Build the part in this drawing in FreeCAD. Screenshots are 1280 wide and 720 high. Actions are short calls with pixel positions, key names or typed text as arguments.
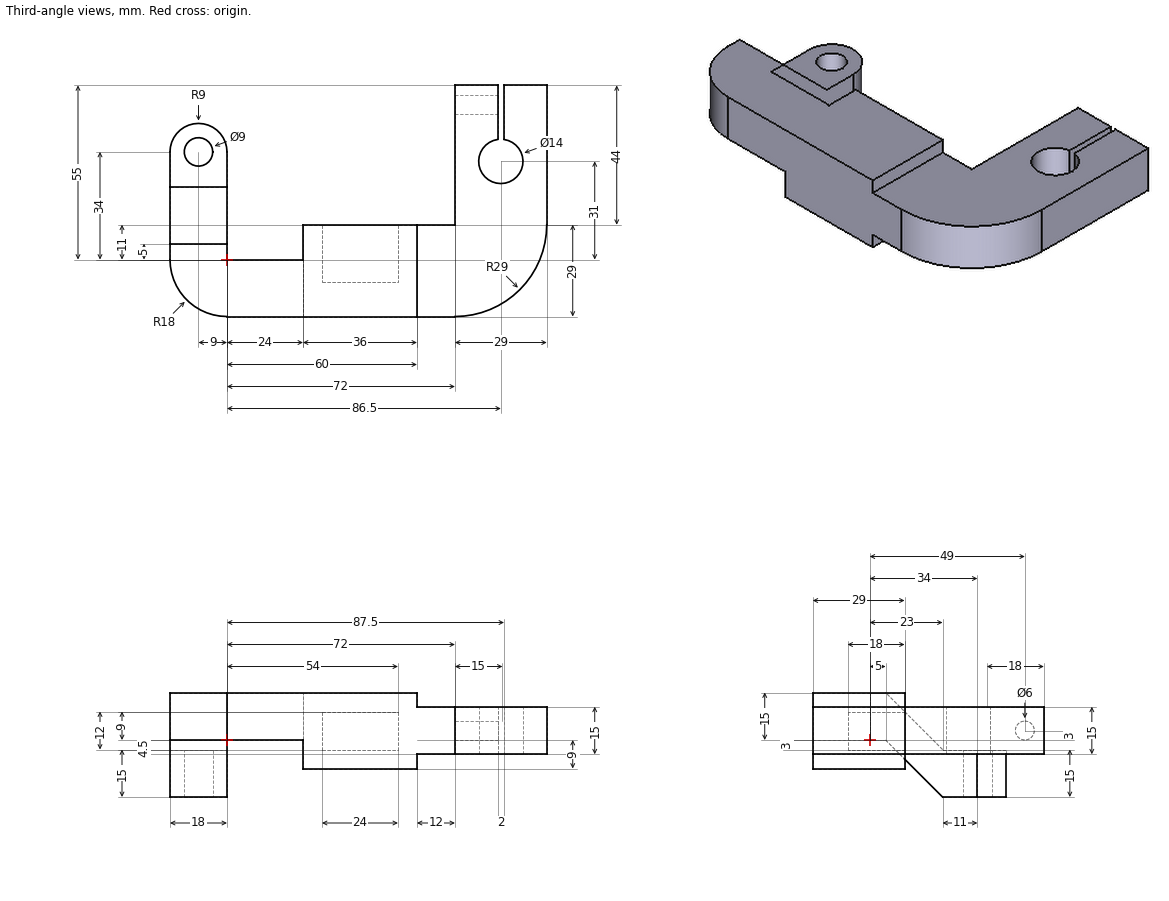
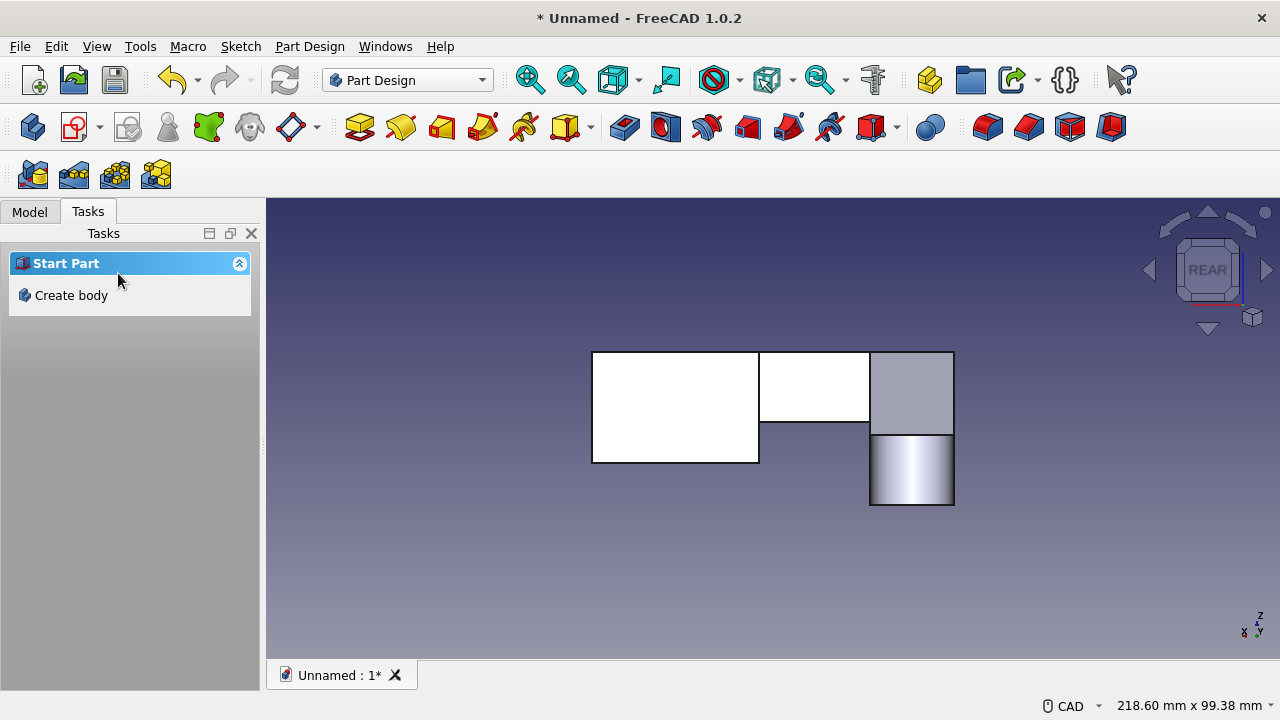
click(531, 80)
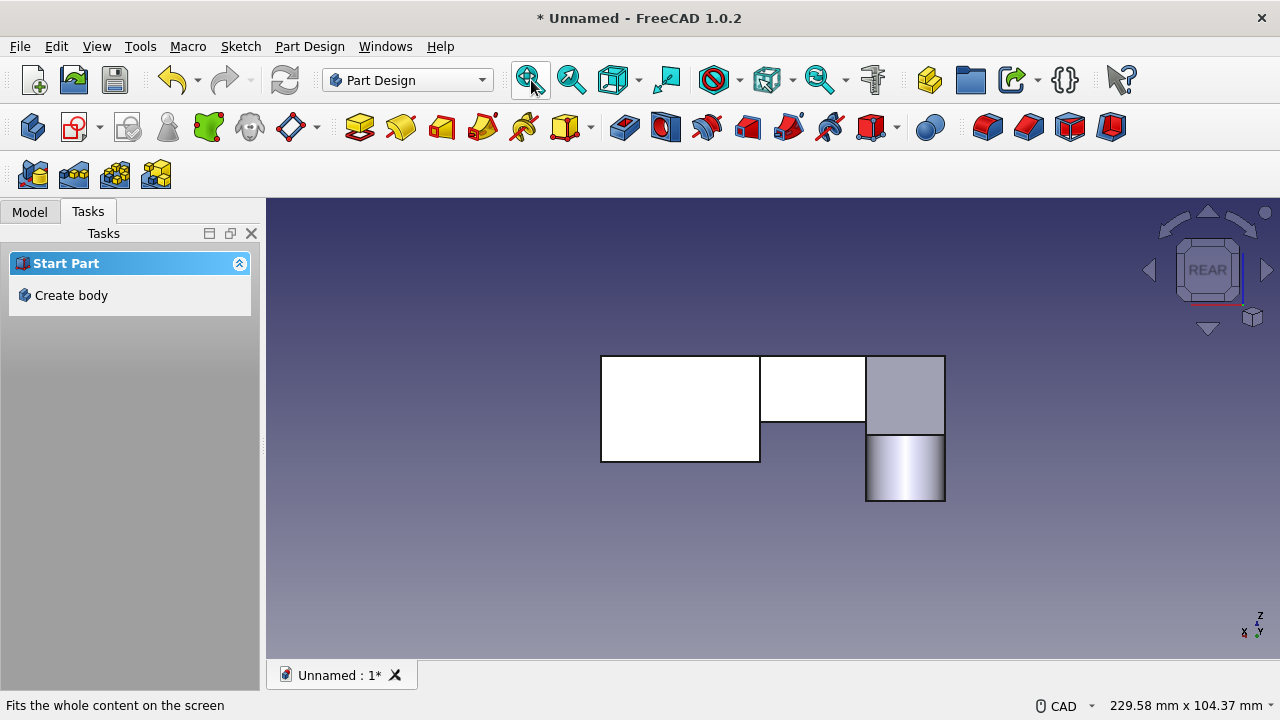
click(658, 408)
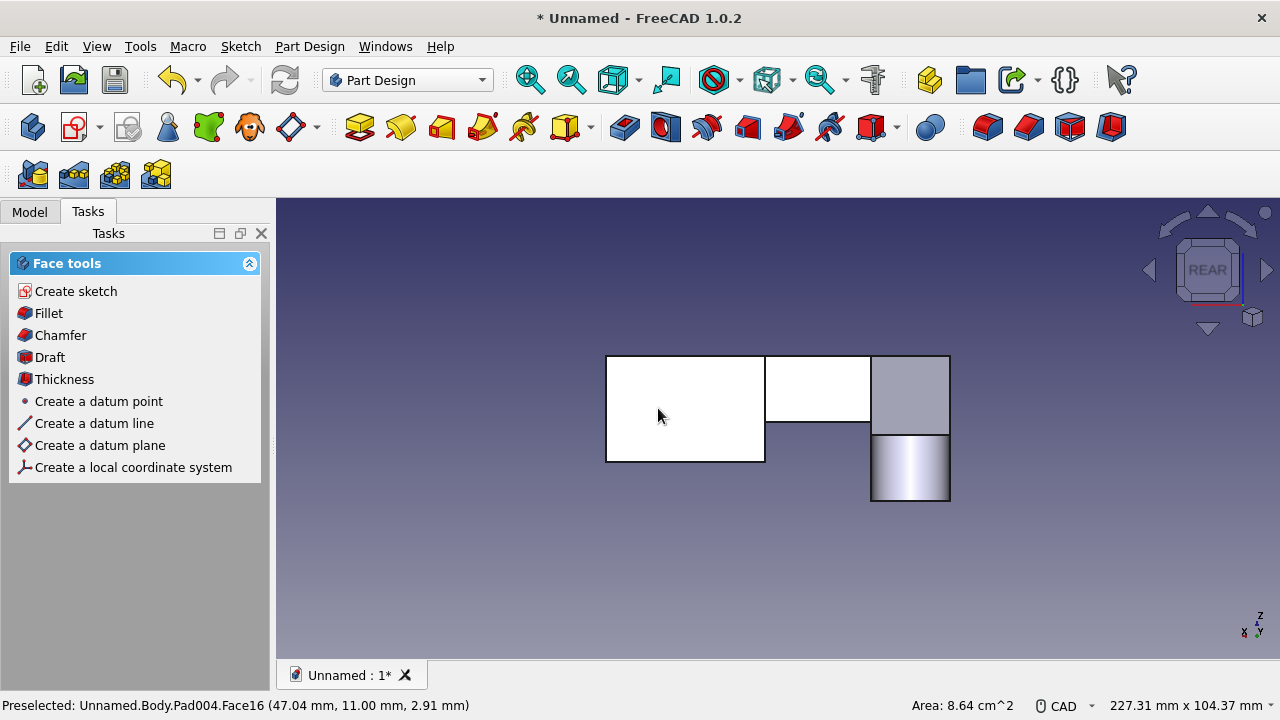
click(74, 128)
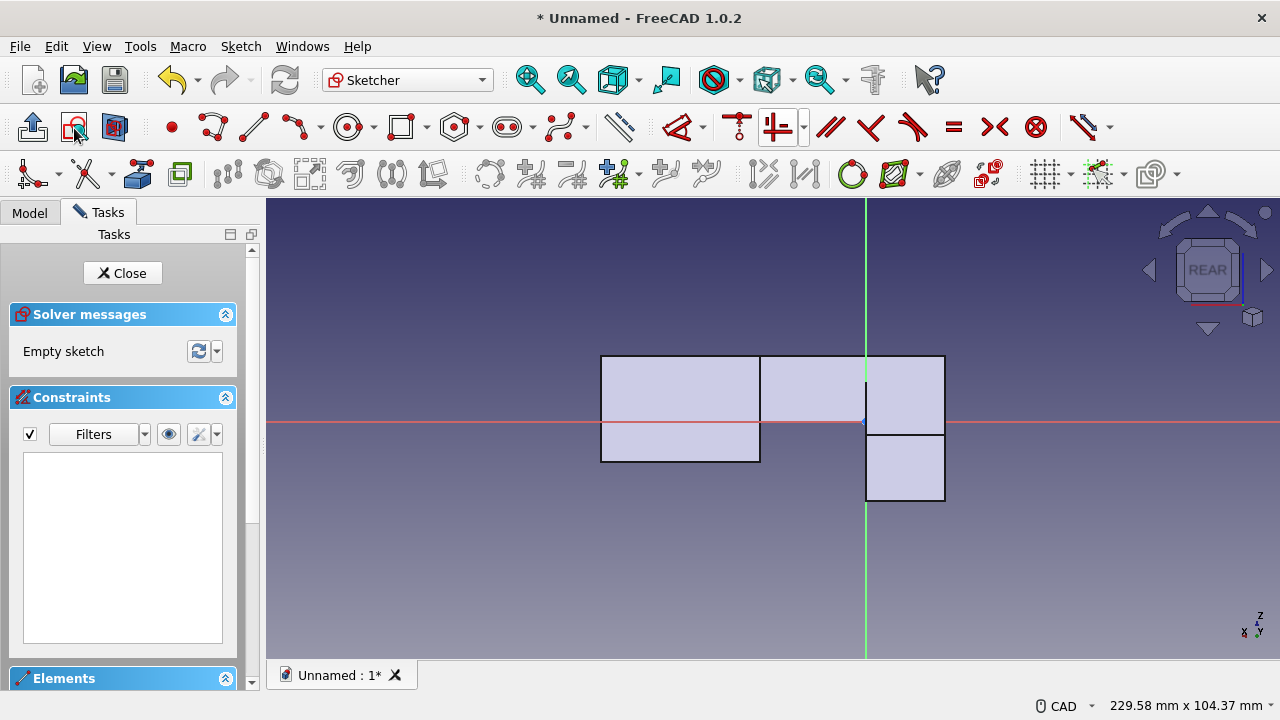
click(115, 128)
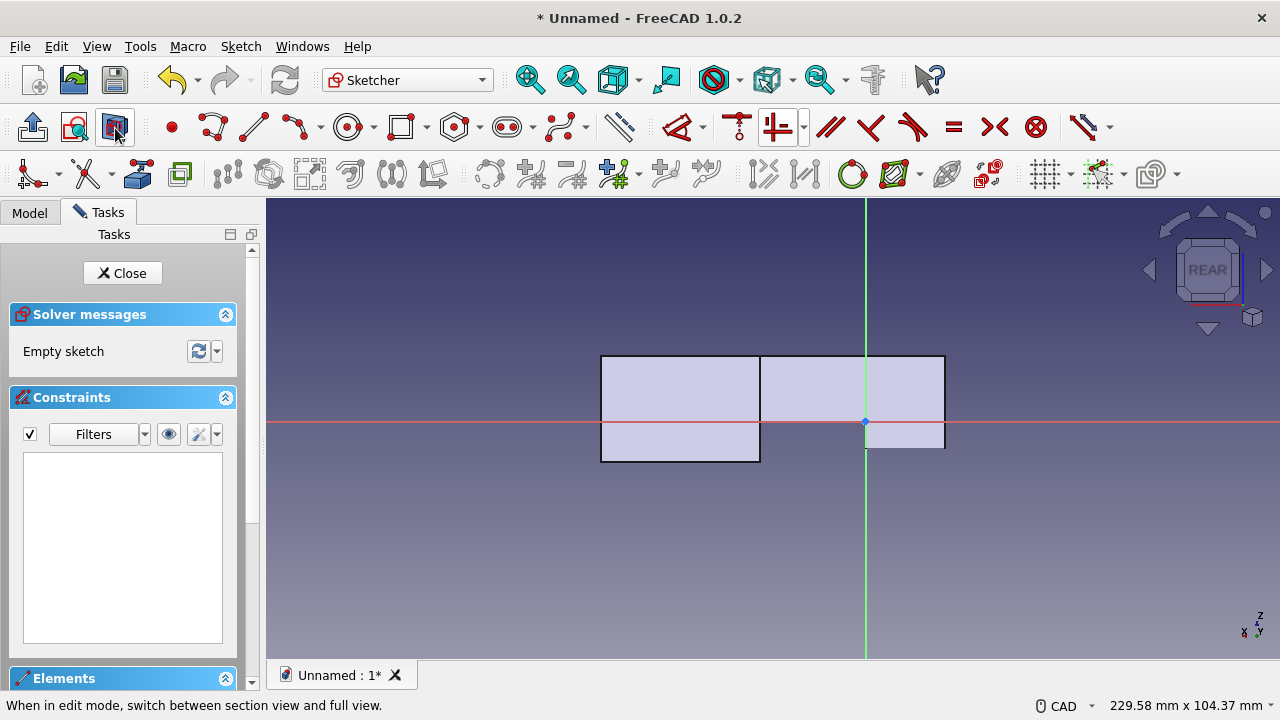
scroll(532, 402, up, 7)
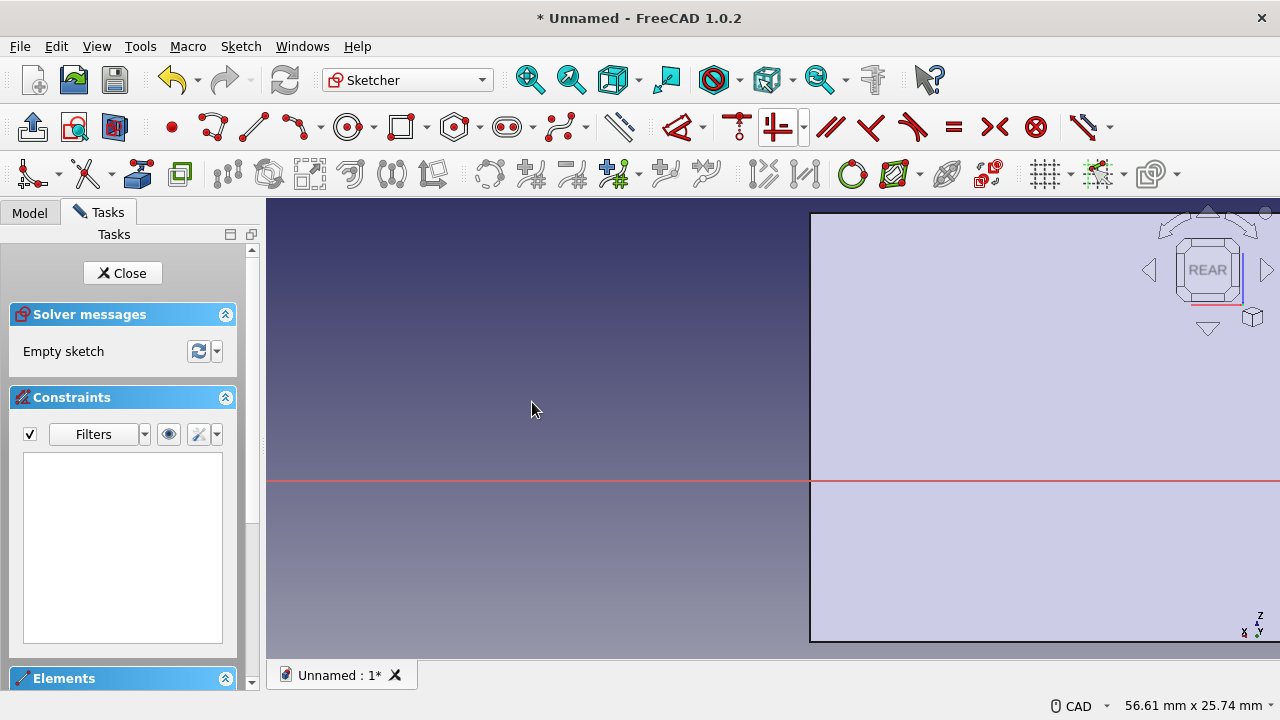
click(400, 128)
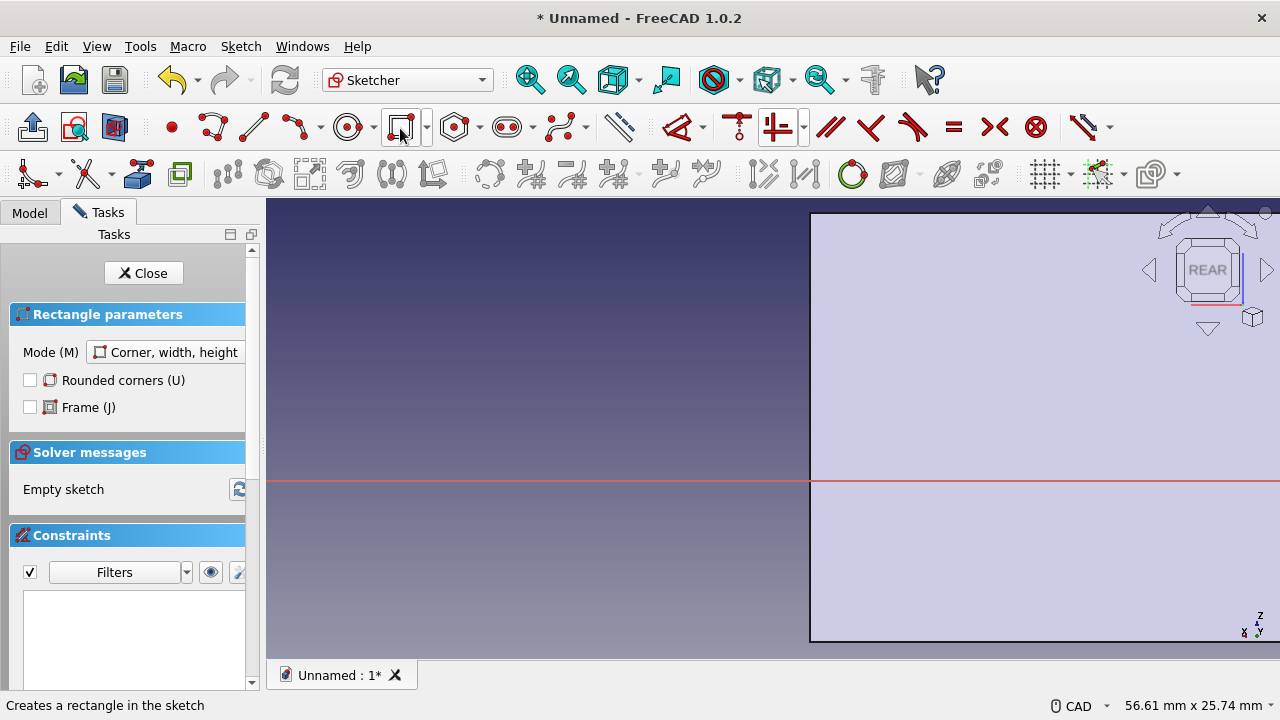
click(595, 293)
move(810, 562)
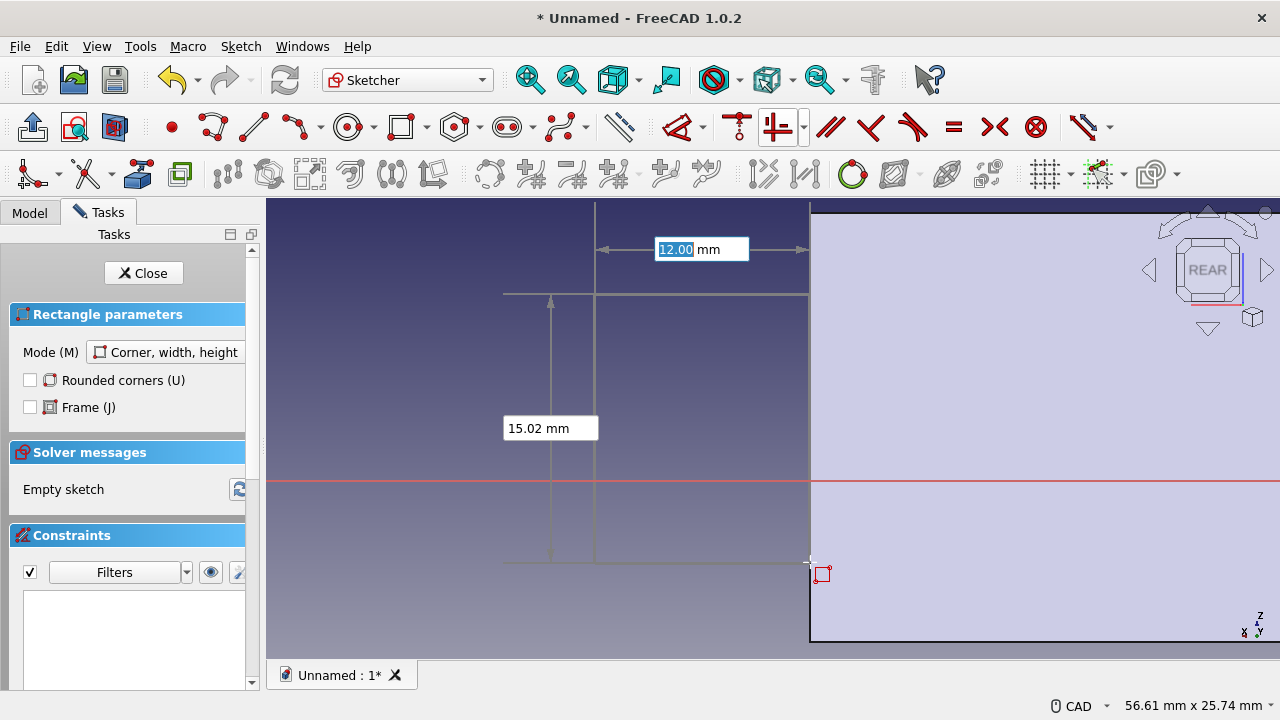
text(12)
key(Tab)
text(15)
key(Return)
key(Escape)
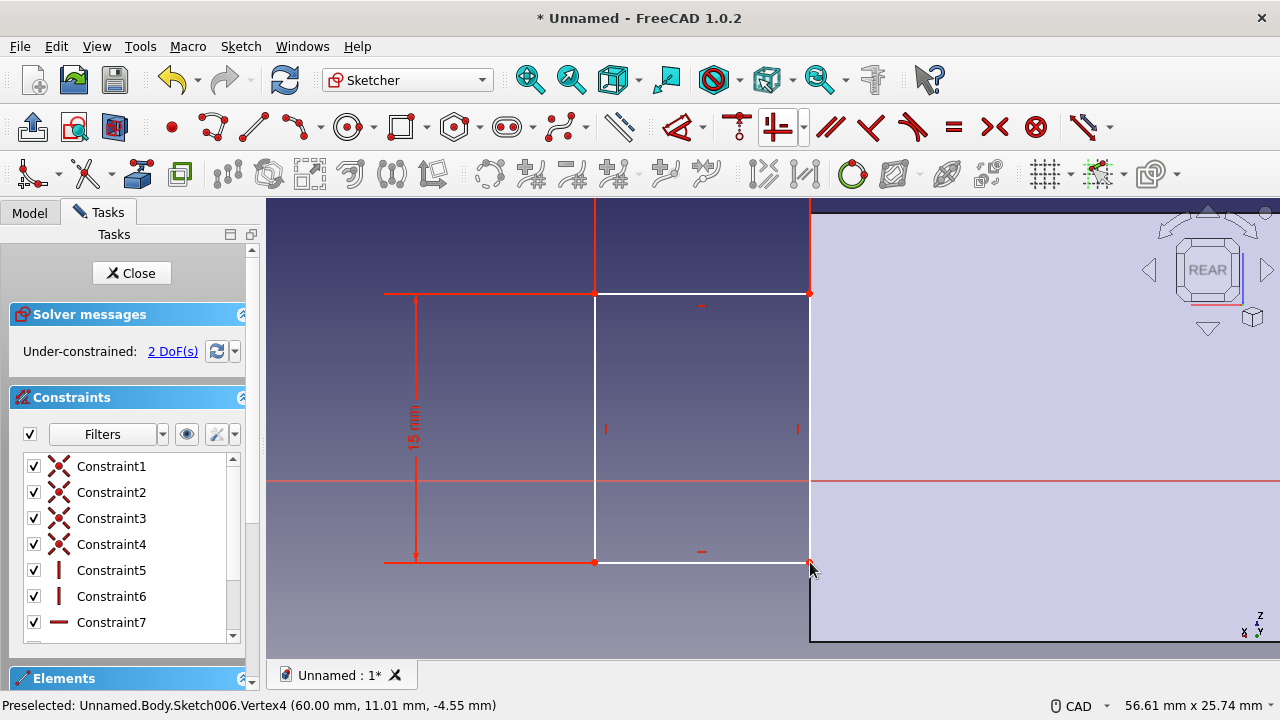
click(676, 128)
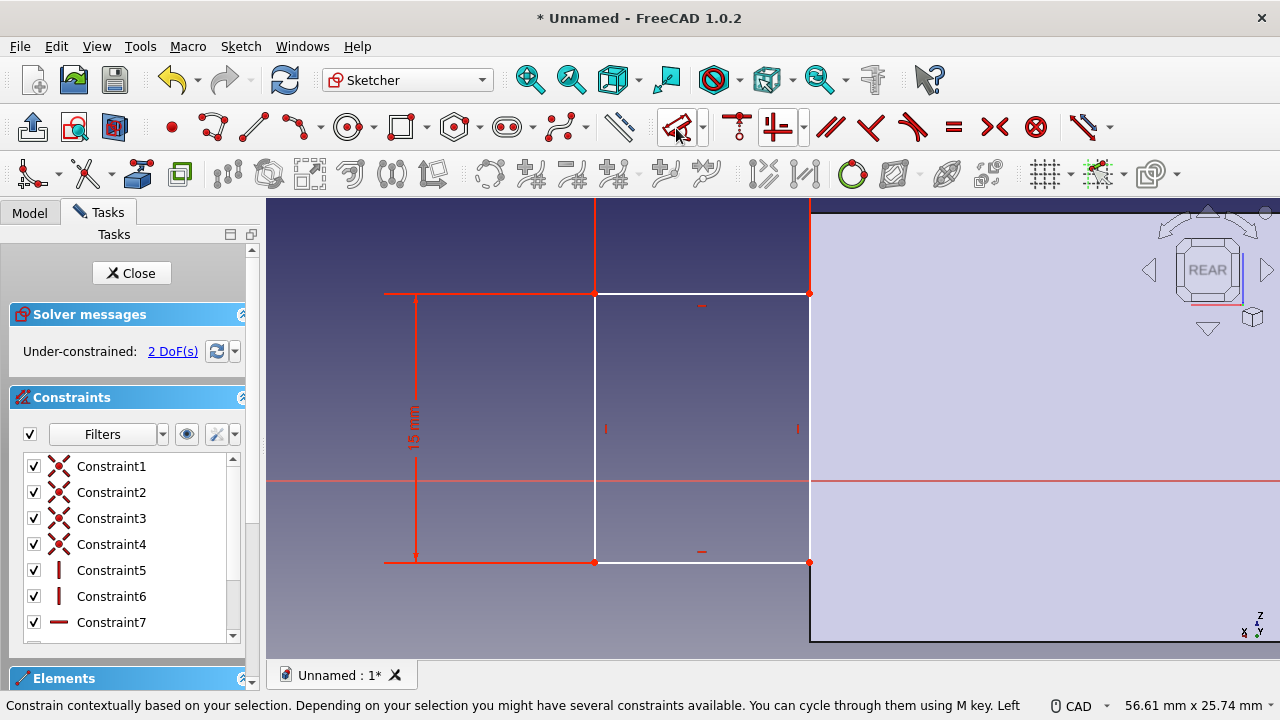
click(595, 294)
click(855, 260)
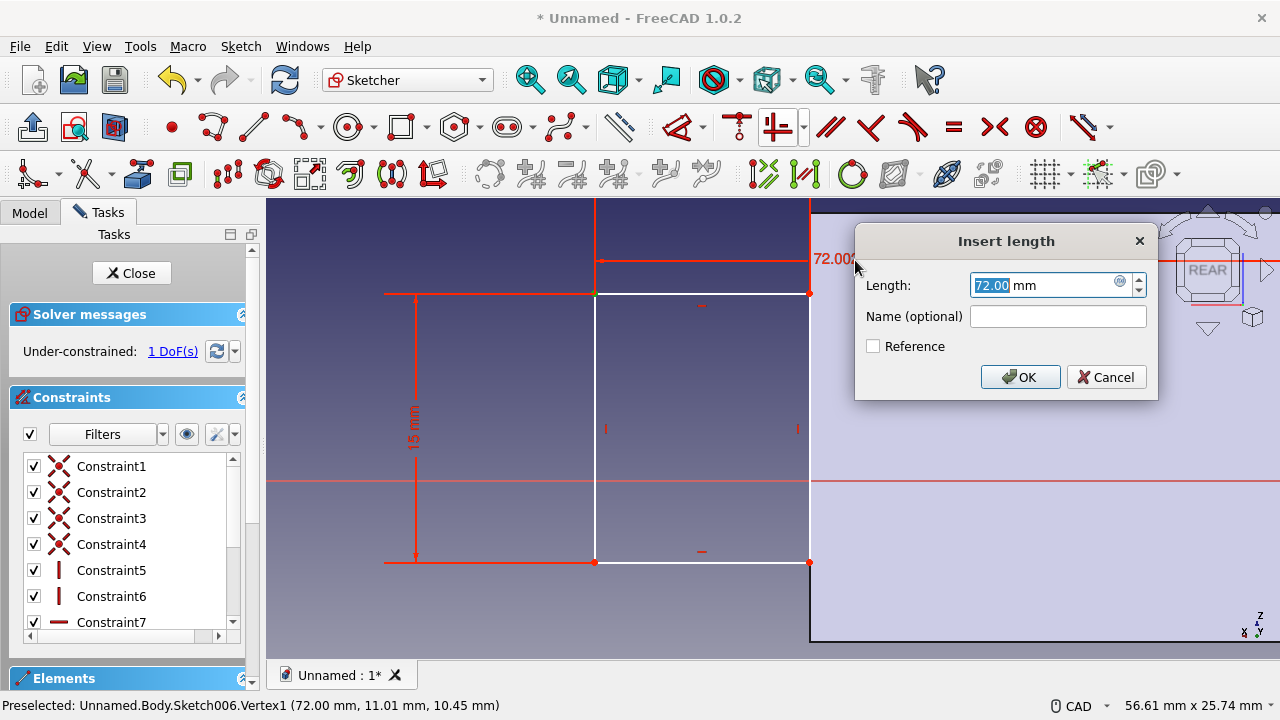
text(72)
key(Return)